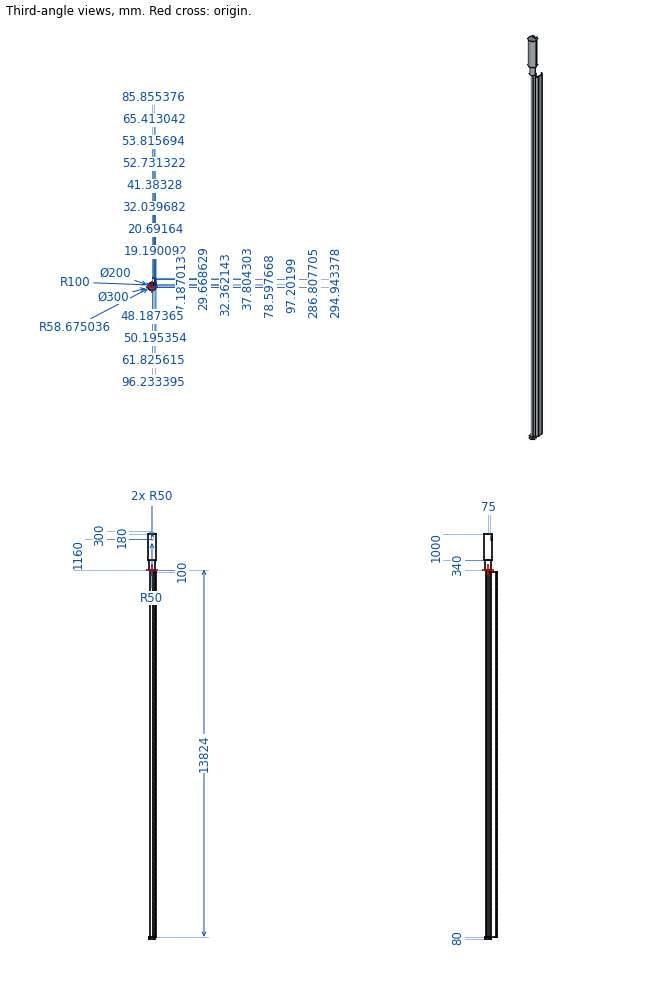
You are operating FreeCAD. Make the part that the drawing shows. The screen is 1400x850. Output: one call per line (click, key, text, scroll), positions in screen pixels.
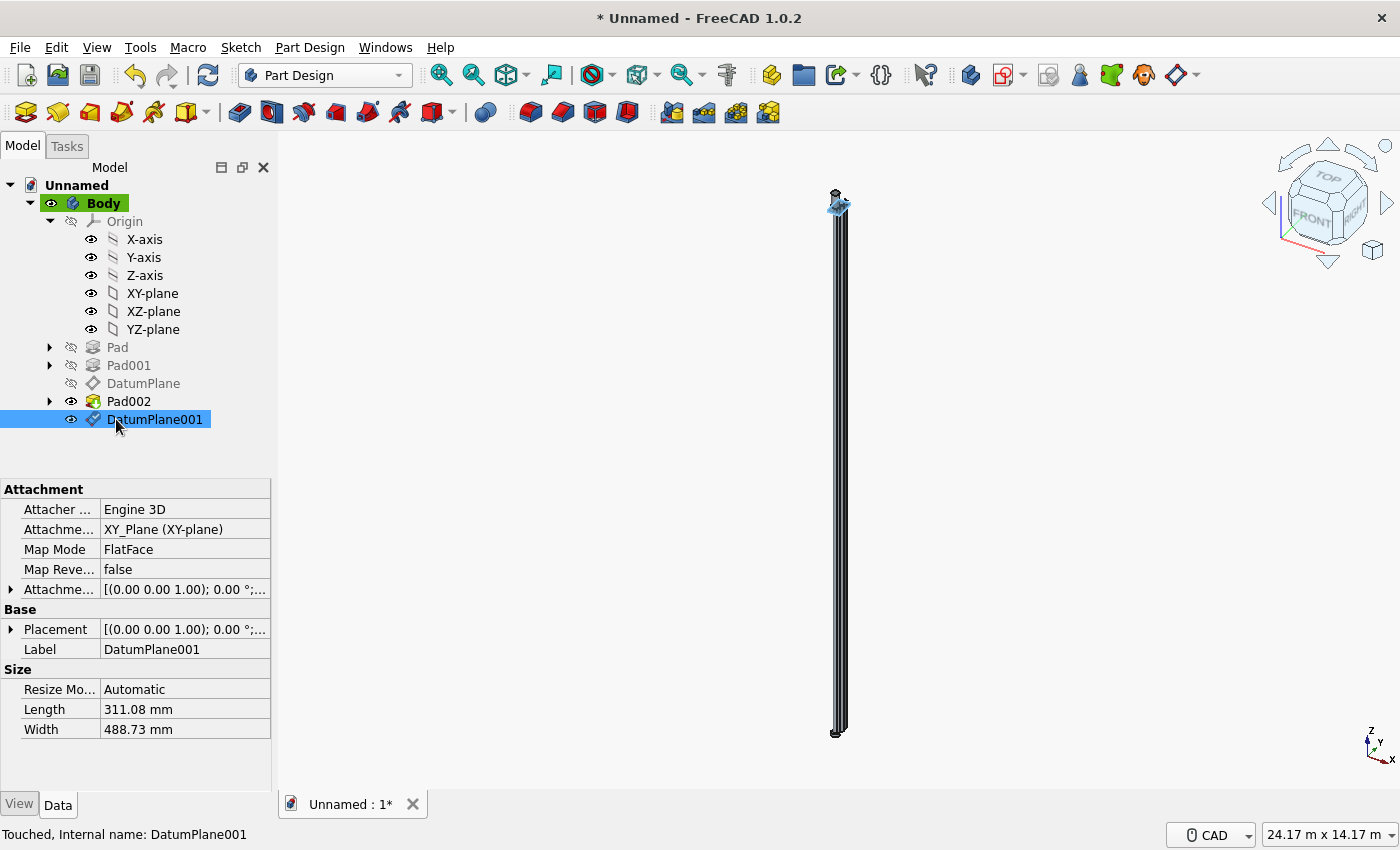
click(1004, 76)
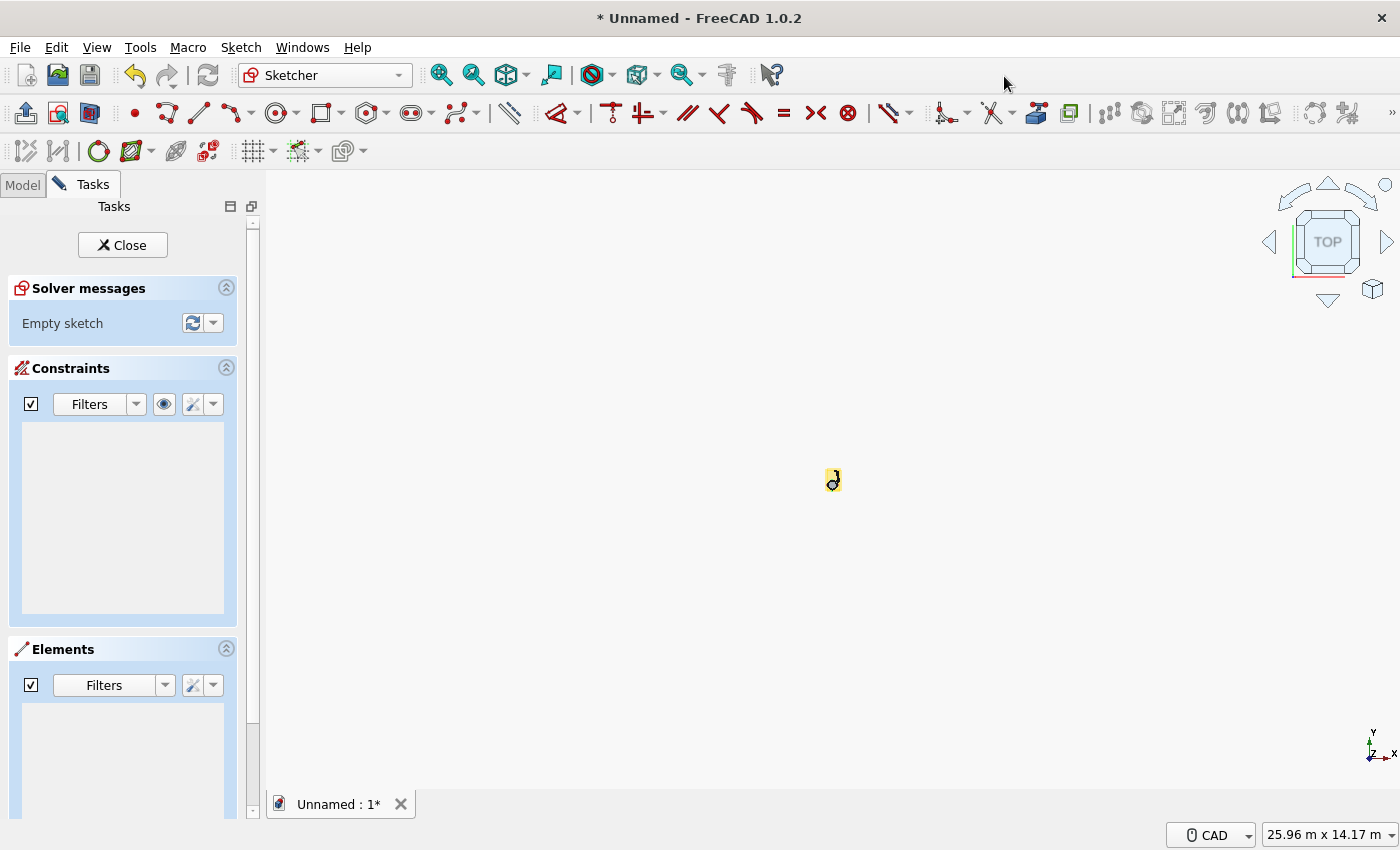
click(90, 114)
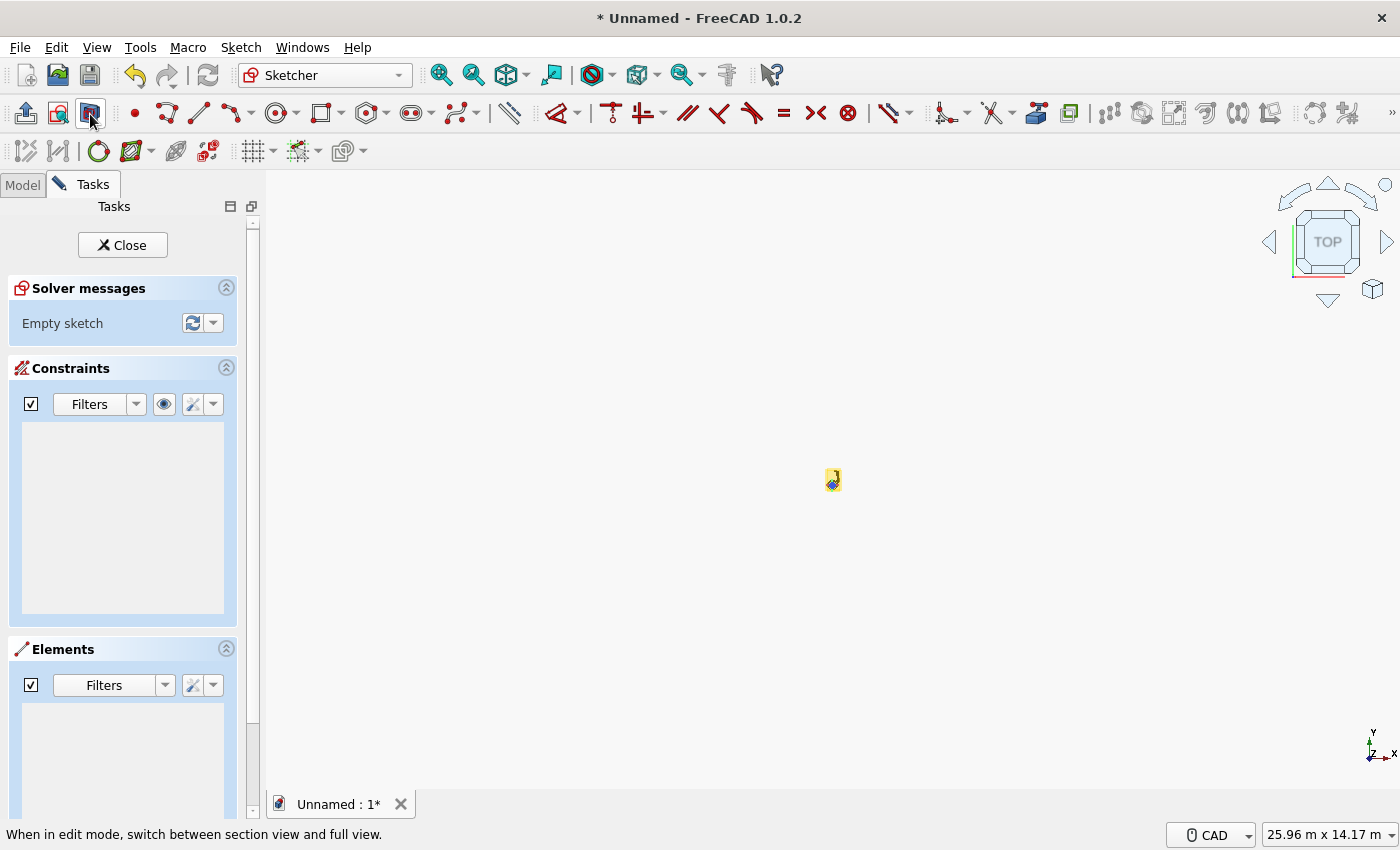
scroll(839, 478, up, 15)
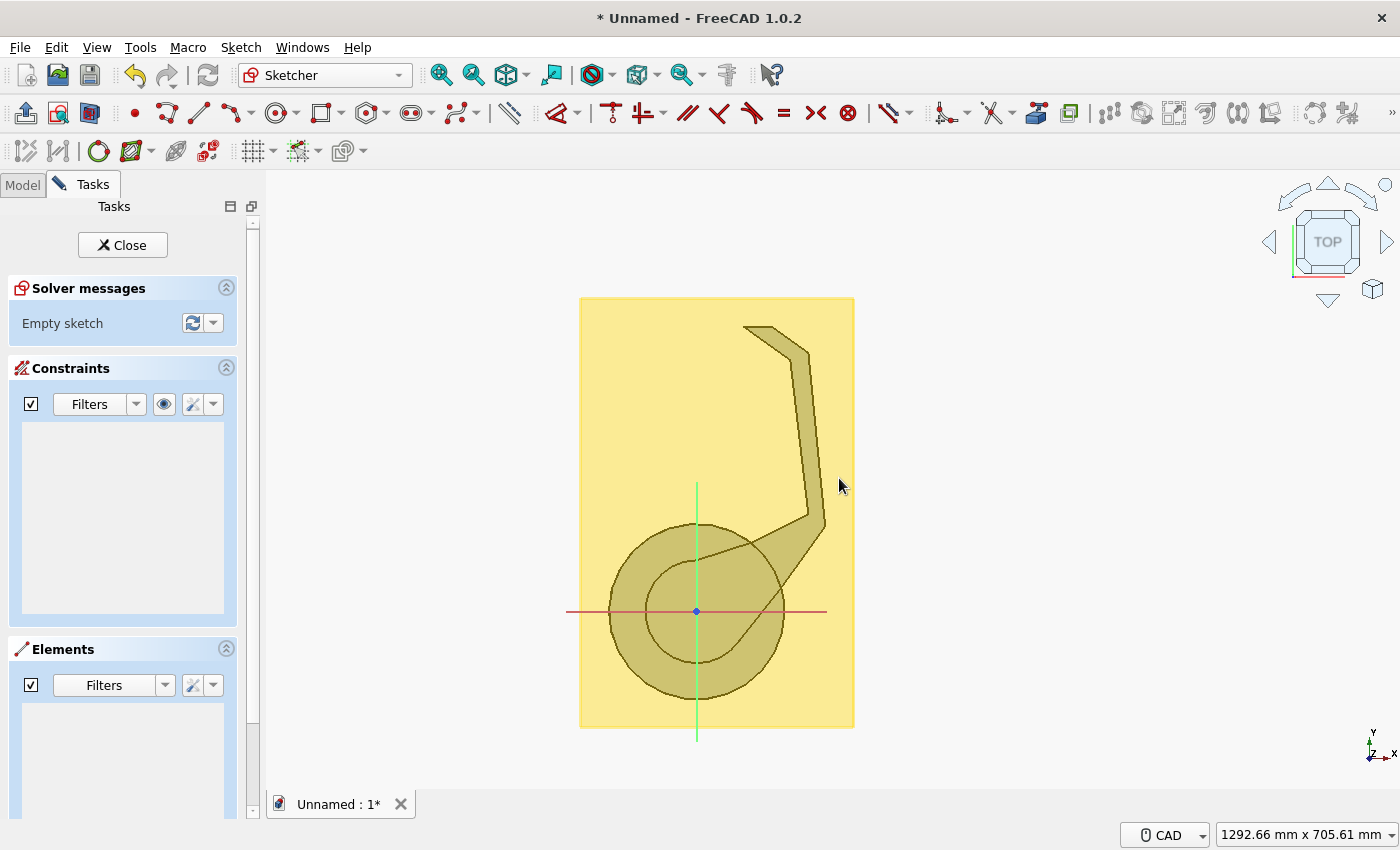
scroll(754, 449, up, 2)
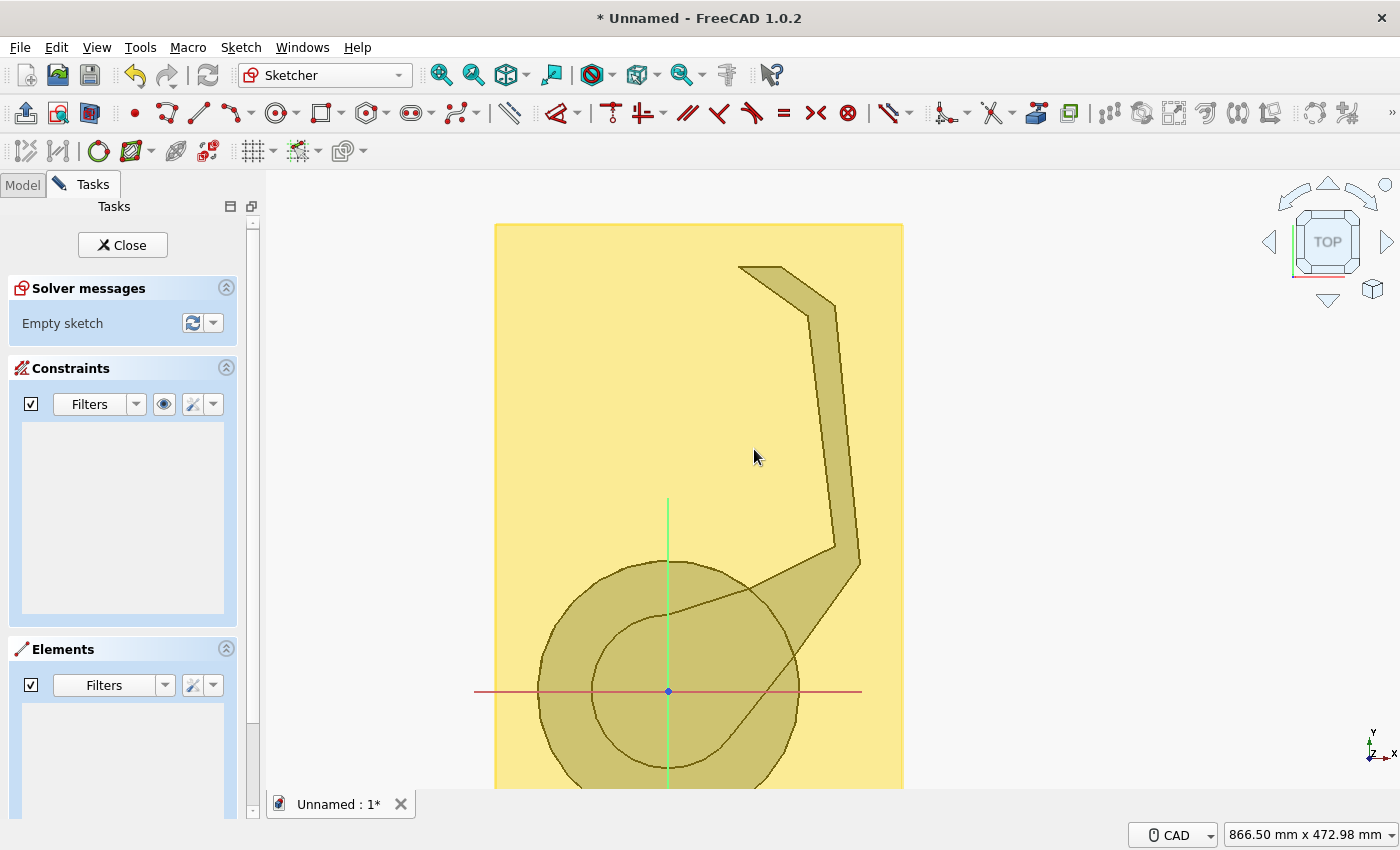
key(g)
key(m)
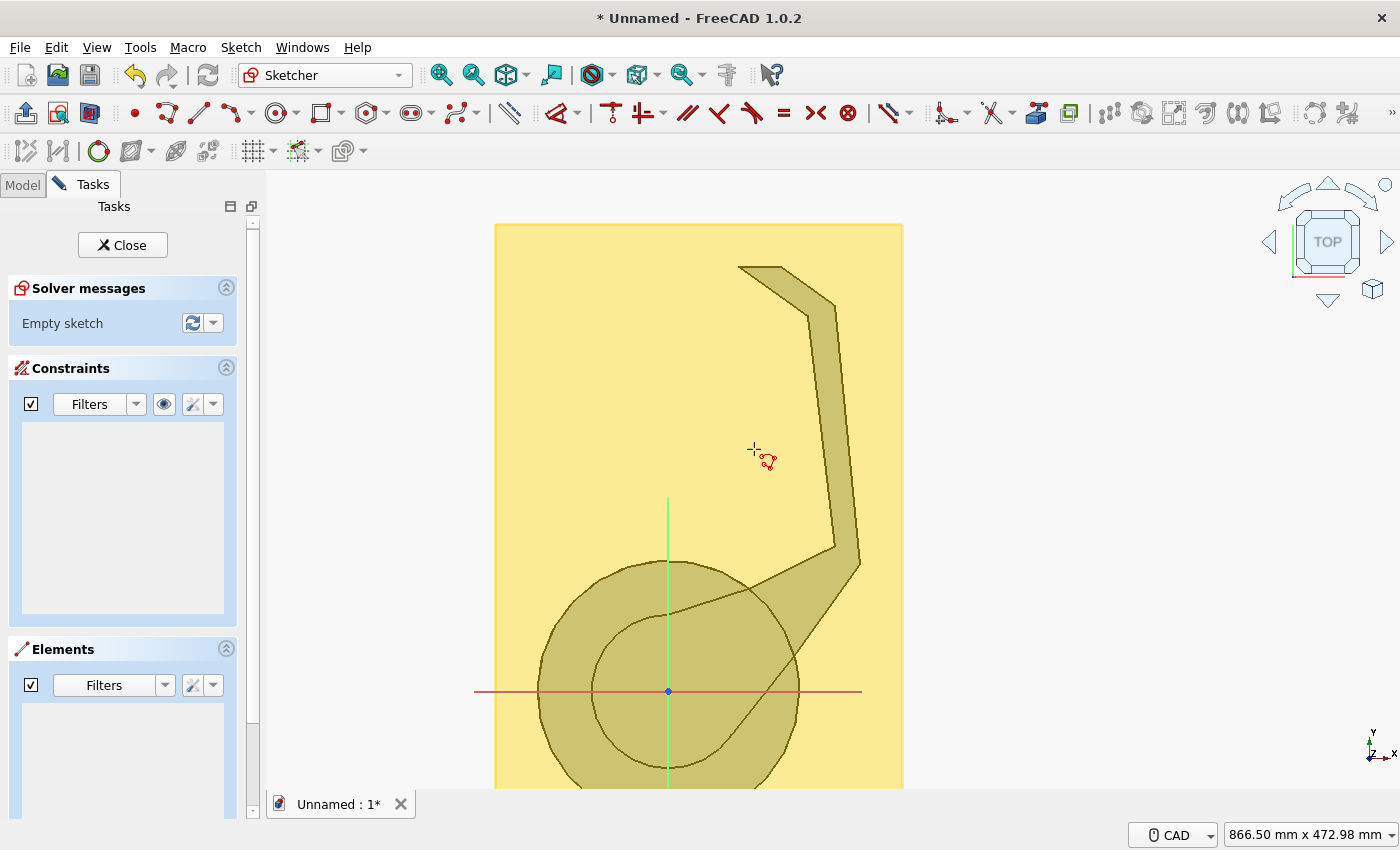
click(794, 656)
click(860, 564)
click(835, 306)
click(781, 267)
click(739, 267)
click(808, 316)
click(835, 546)
click(749, 589)
right_click(749, 589)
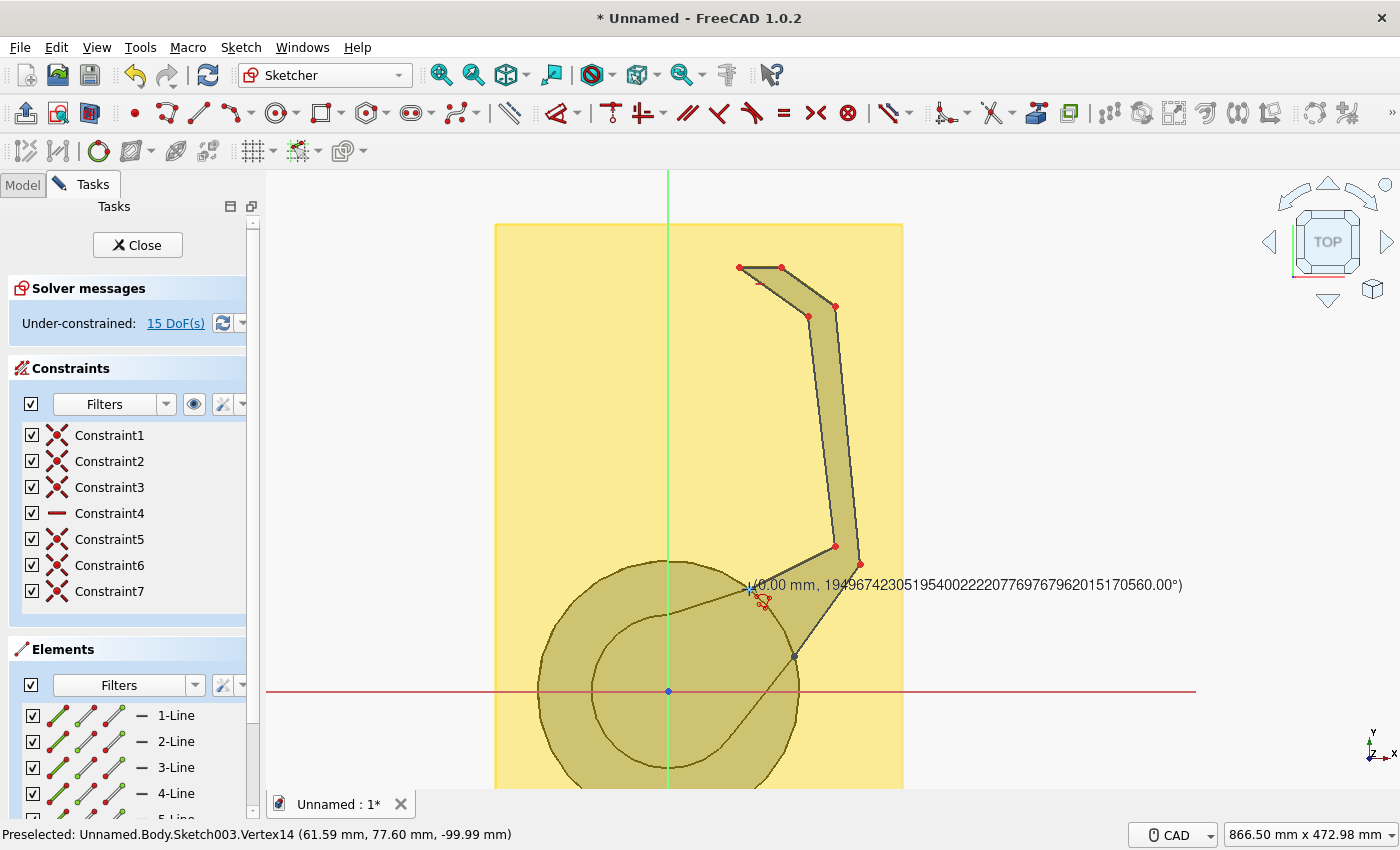
click(232, 114)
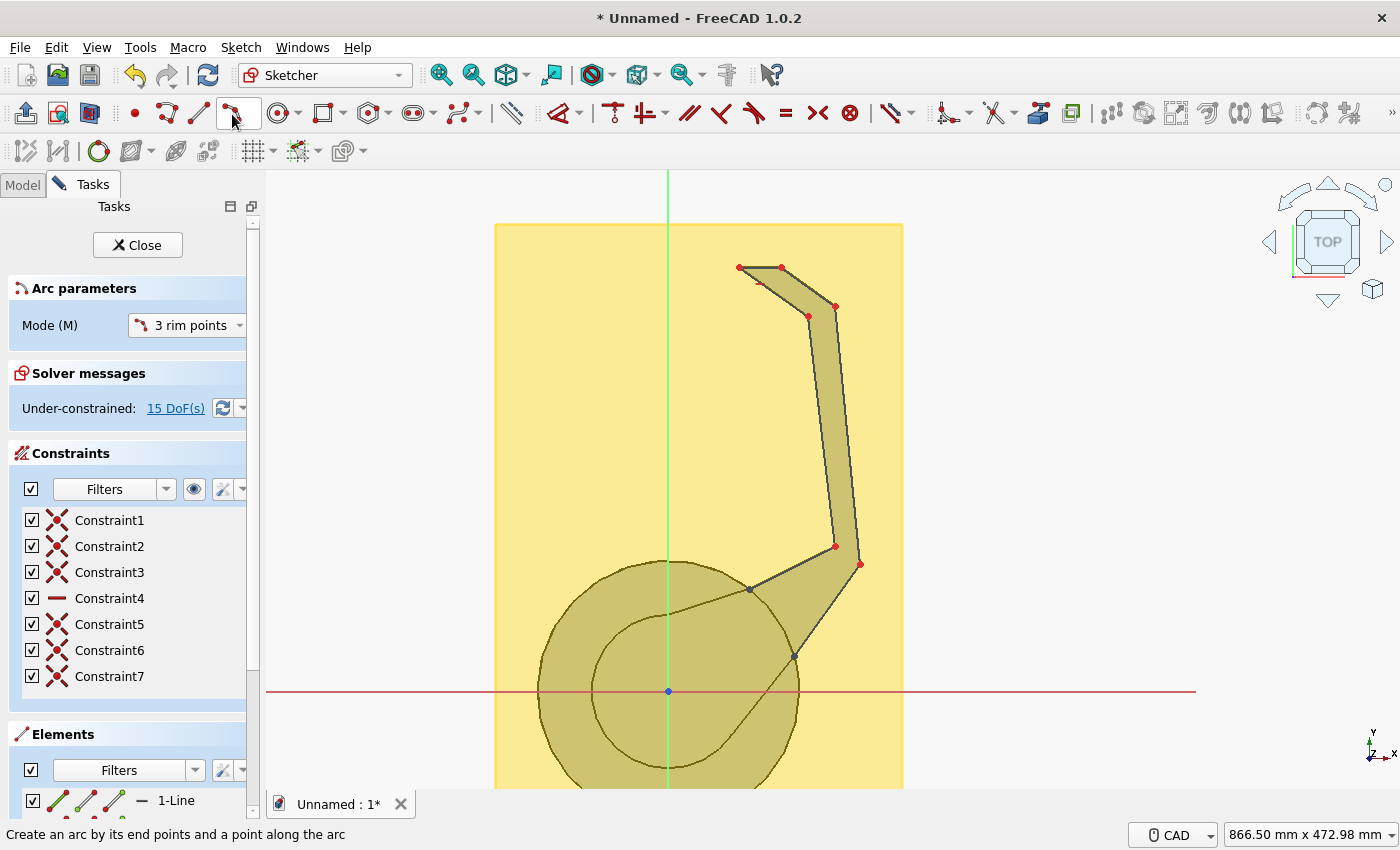
click(749, 590)
click(794, 657)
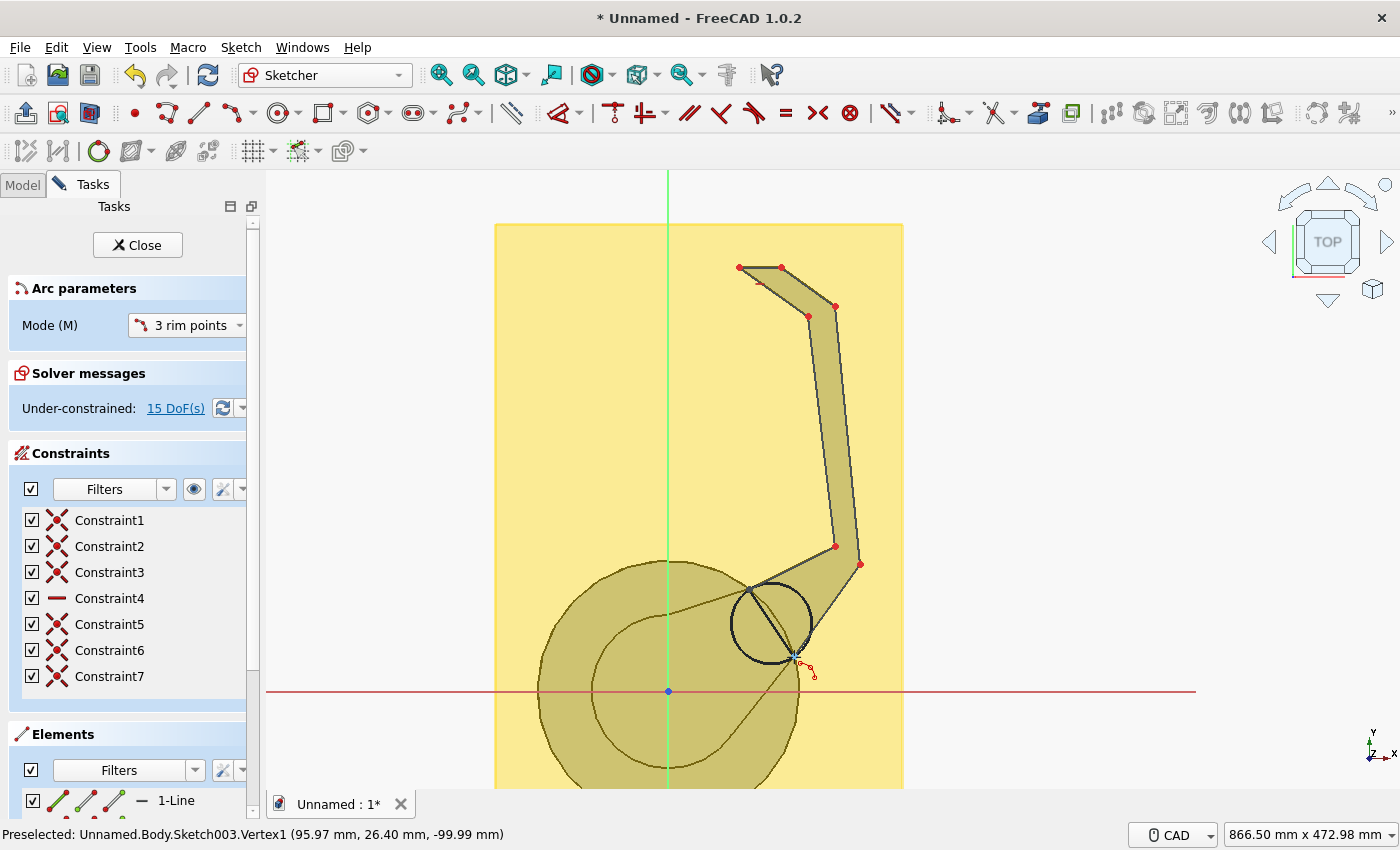
scroll(777, 619, up, 5)